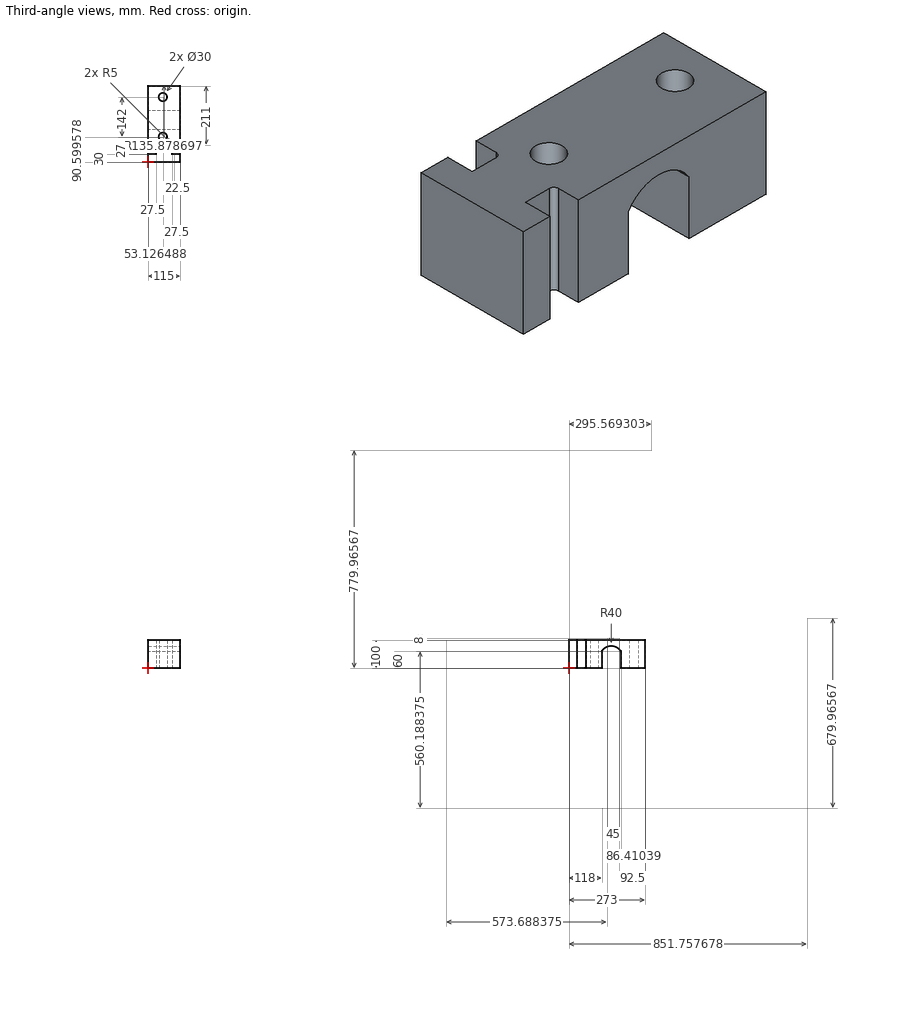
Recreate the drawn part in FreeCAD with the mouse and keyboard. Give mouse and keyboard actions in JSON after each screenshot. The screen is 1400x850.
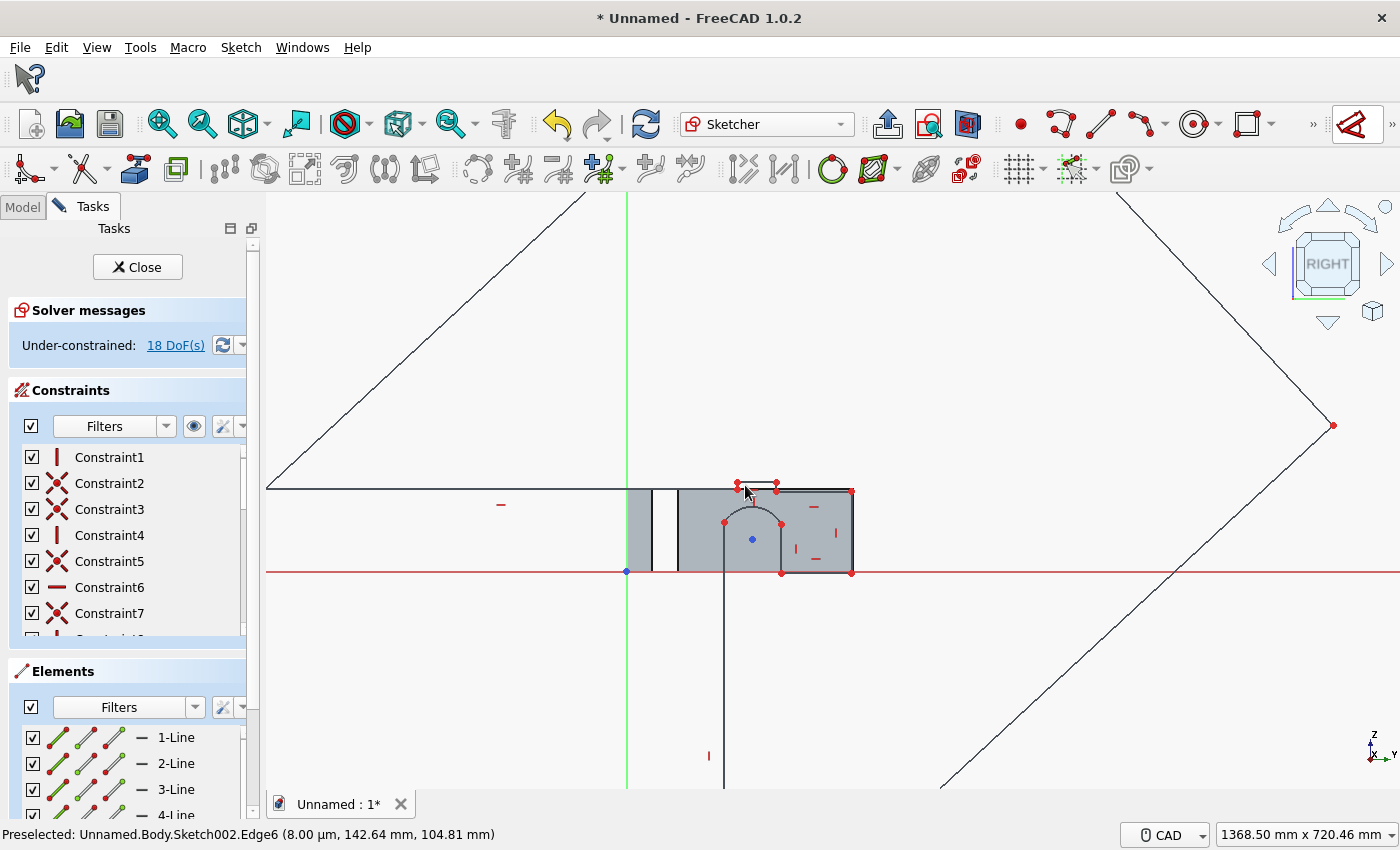
{"action": "key", "text": "d"}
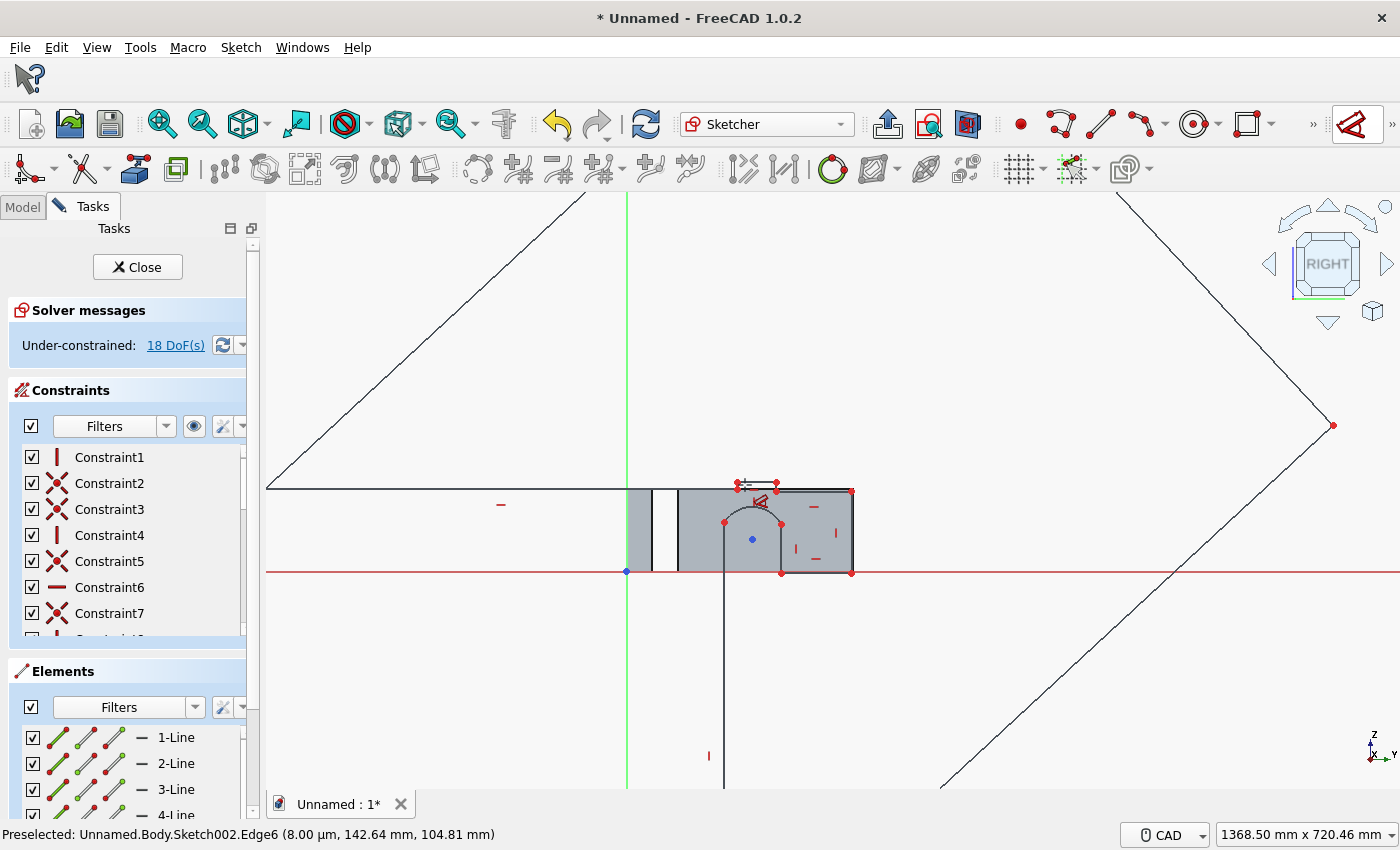
{"action": "left_click", "coordinate": [766, 510]}
{"action": "left_click", "coordinate": [816, 531]}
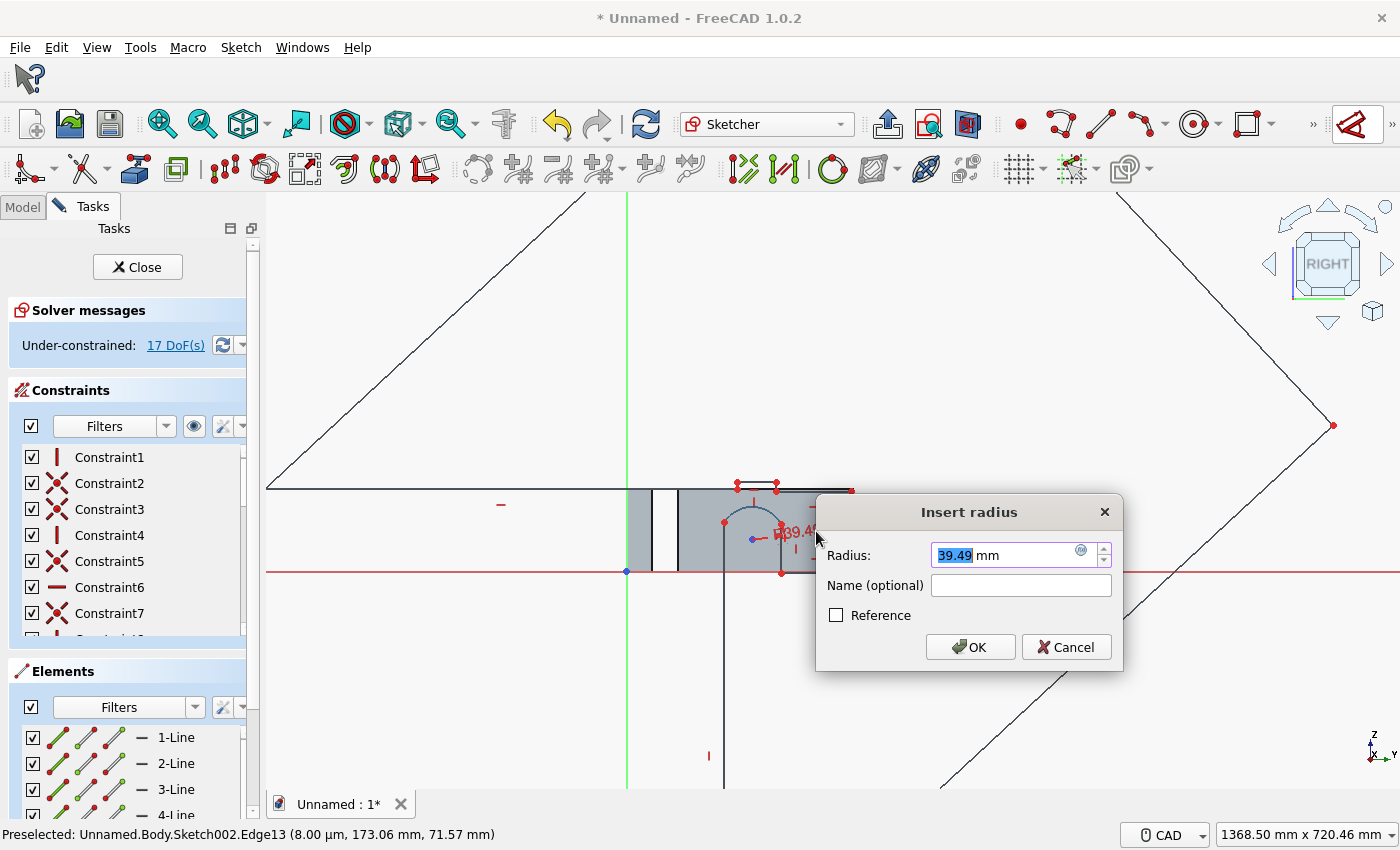
{"action": "type", "text": "40"}
{"action": "key", "text": "Return"}
{"action": "key", "text": "Escape"}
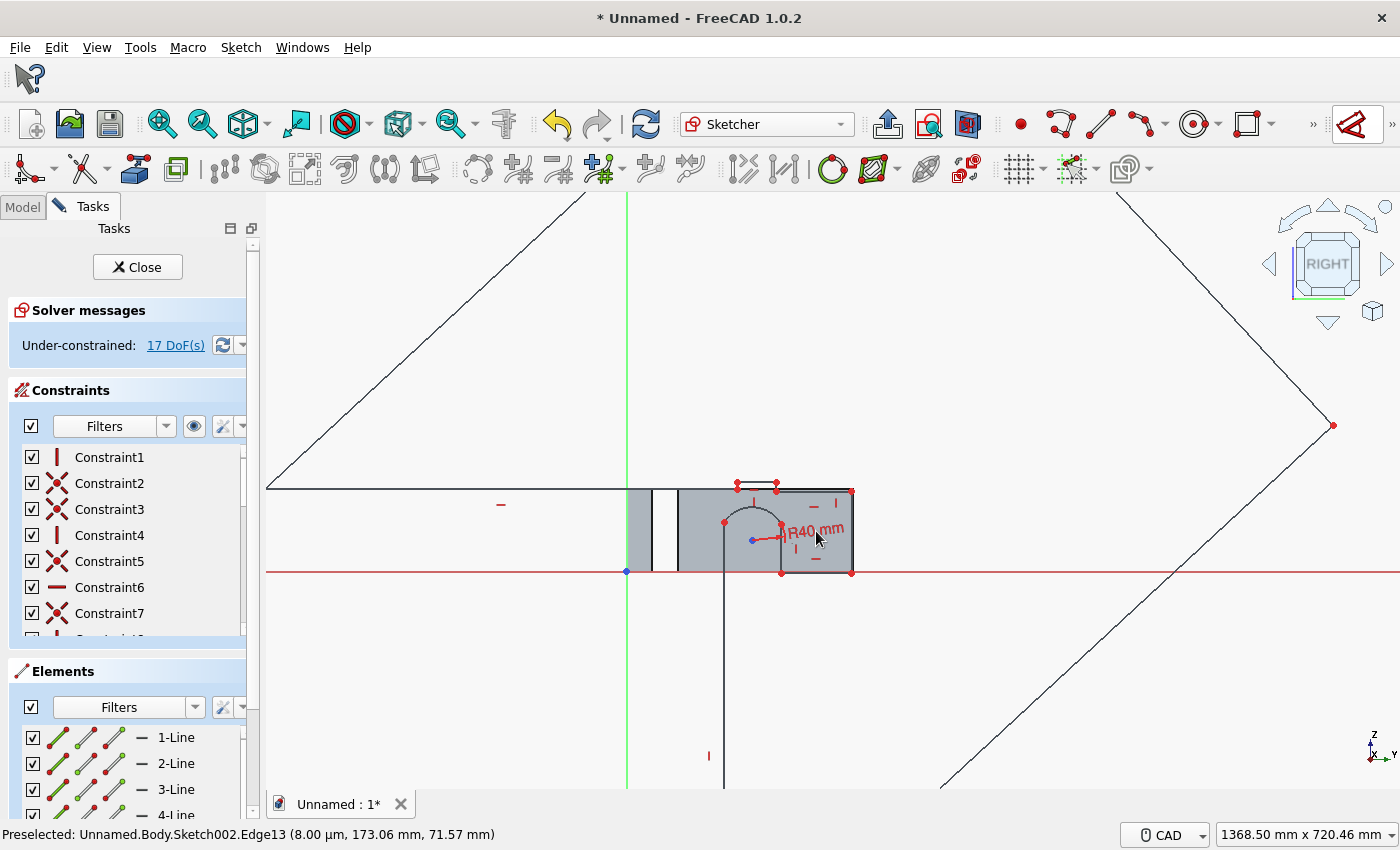
{"action": "left_click", "coordinate": [781, 573]}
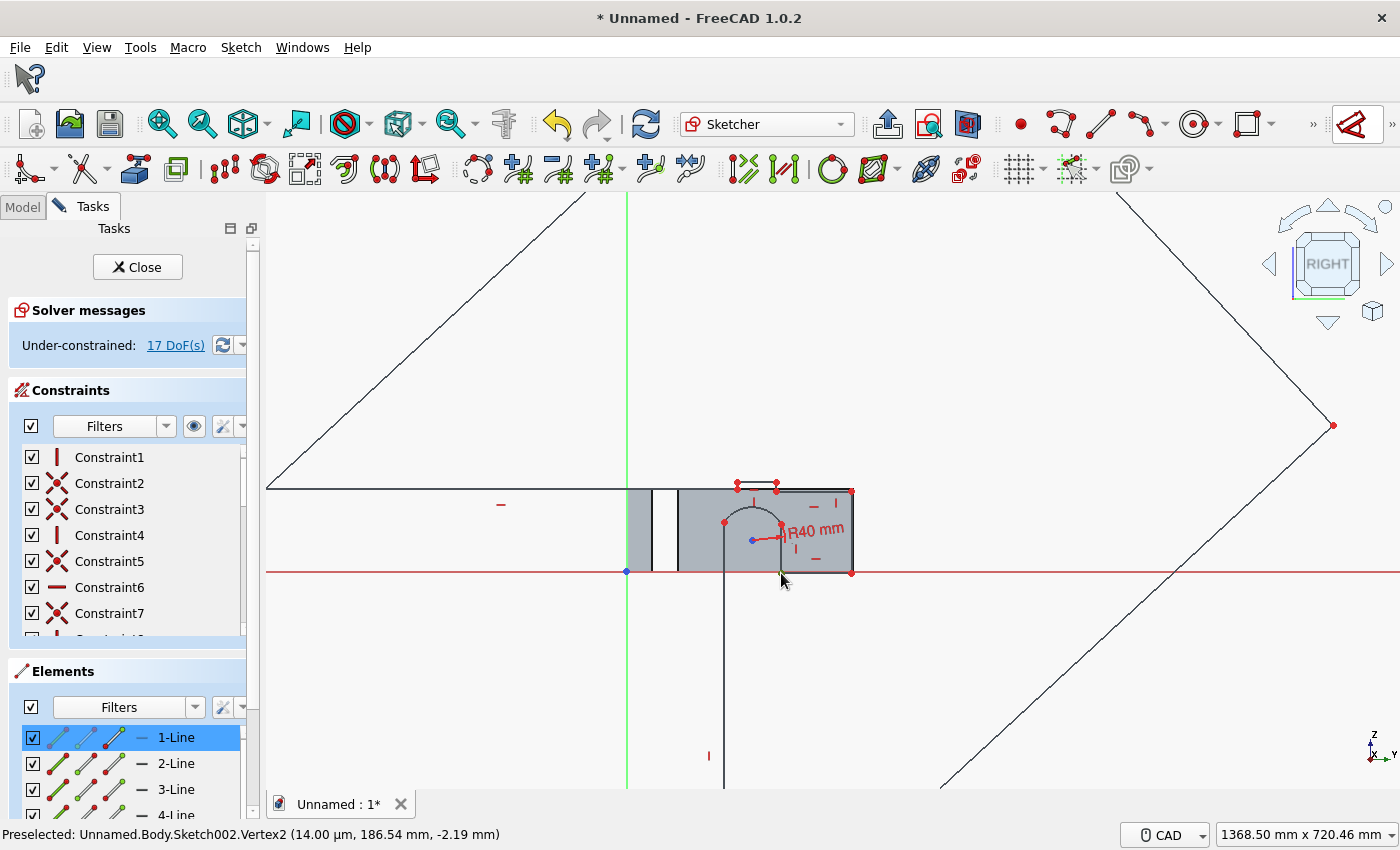
{"action": "left_click", "coordinate": [361, 572]}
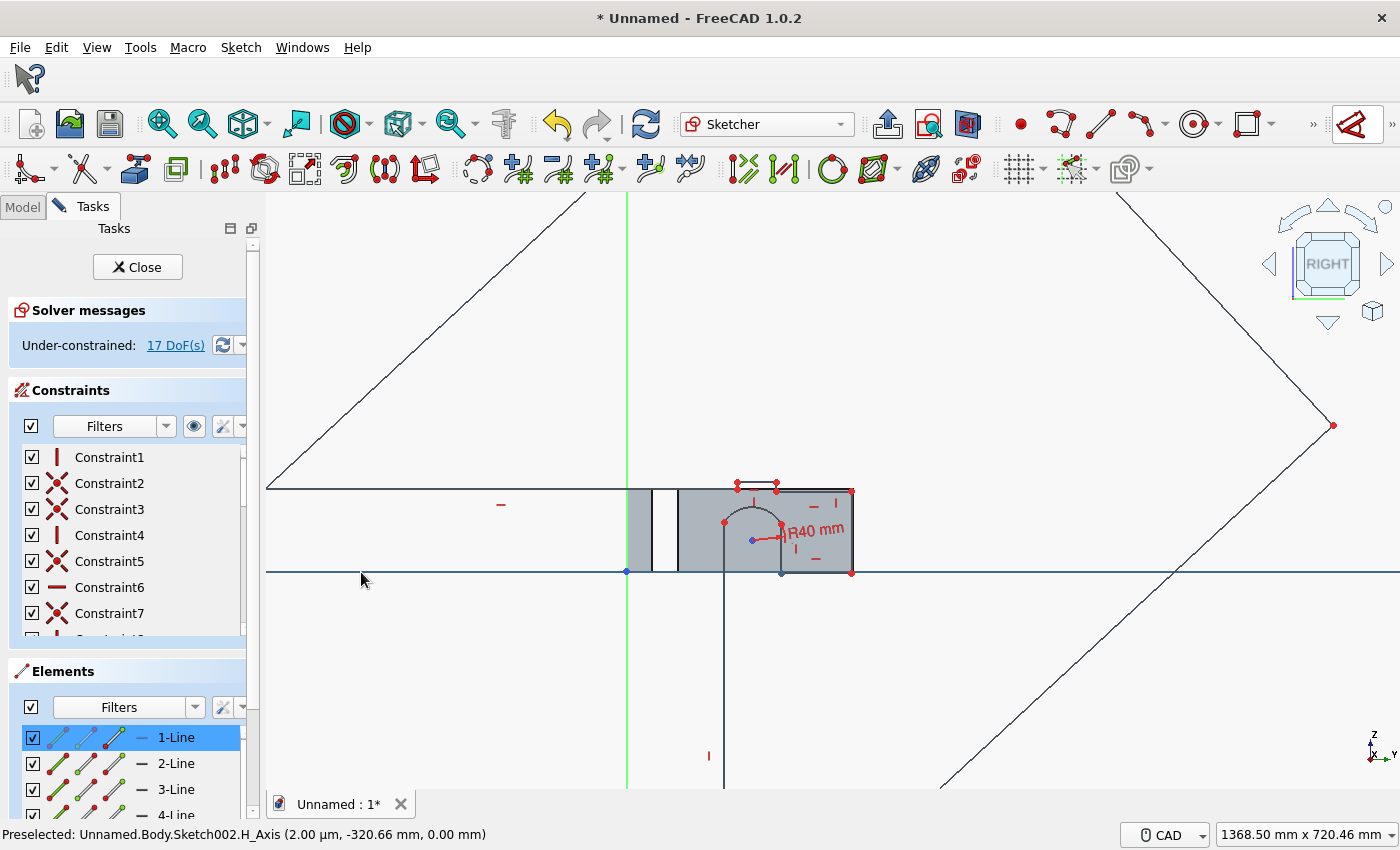
{"action": "key", "text": "c"}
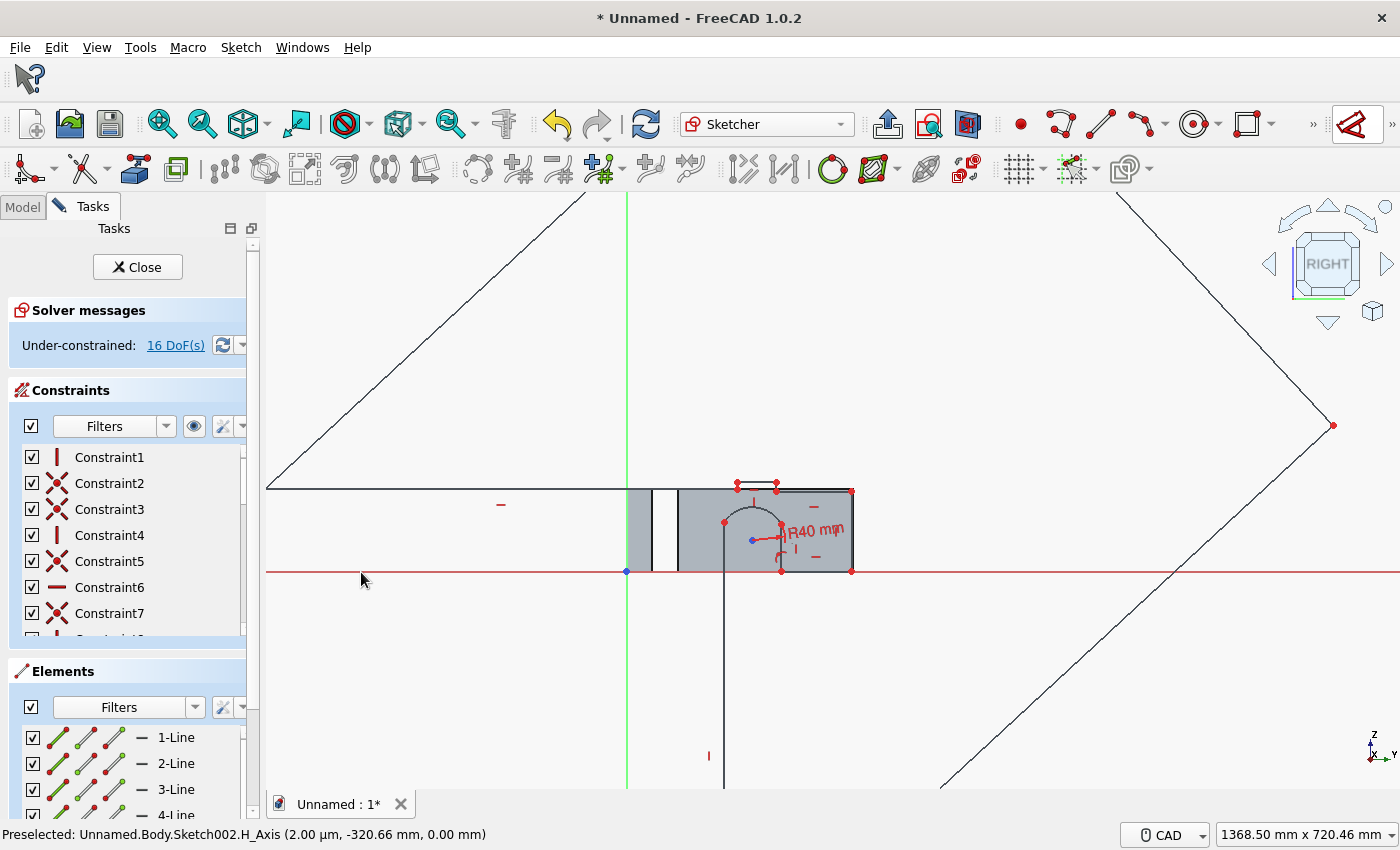
{"action": "left_click", "coordinate": [1352, 124]}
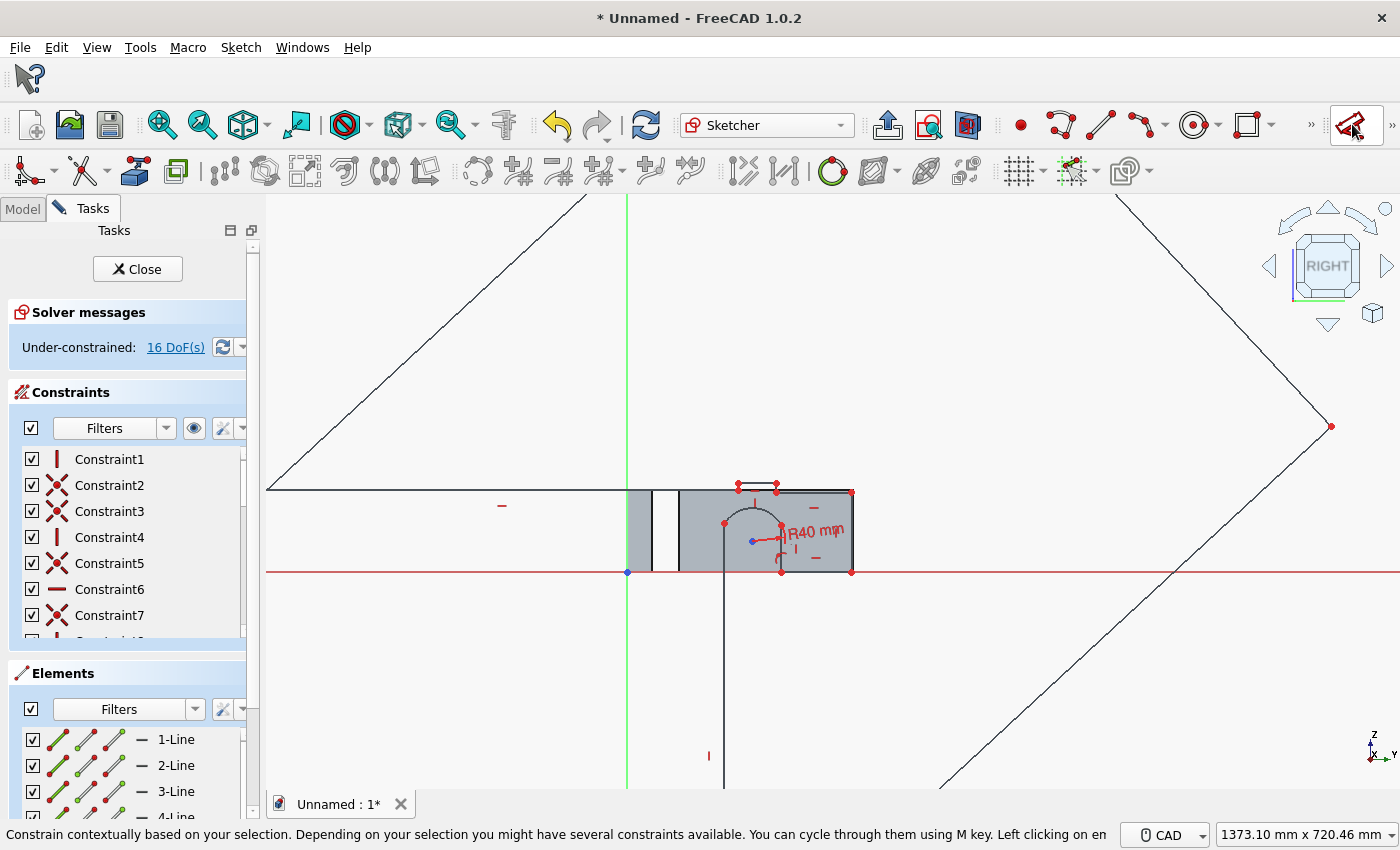
{"action": "scroll", "coordinate": [776, 488], "scroll_direction": "up", "scroll_amount": 9}